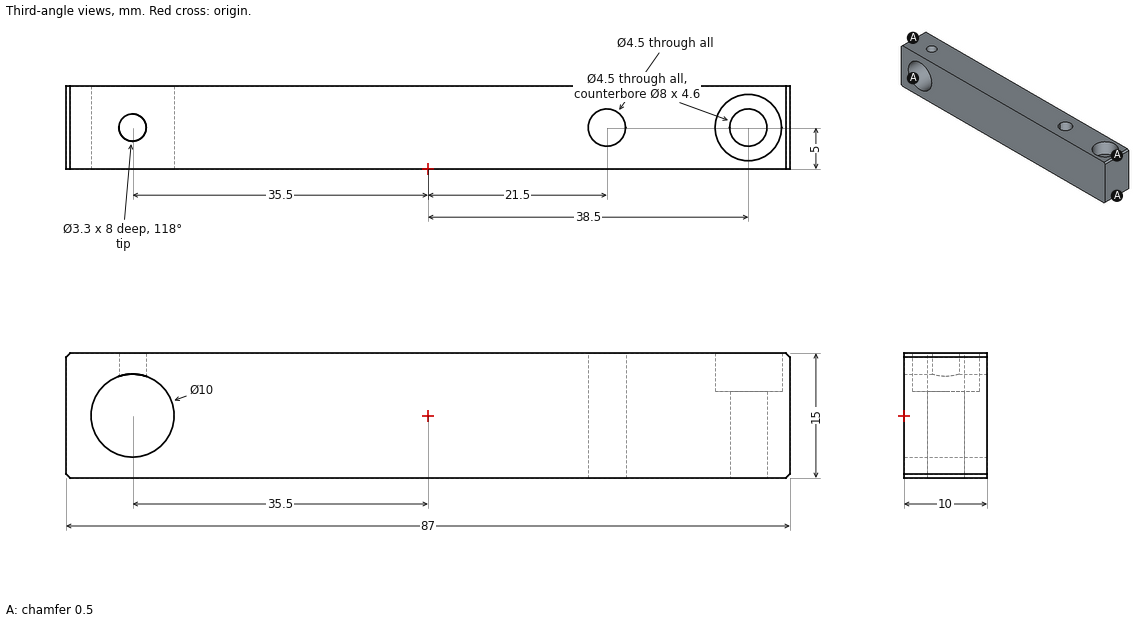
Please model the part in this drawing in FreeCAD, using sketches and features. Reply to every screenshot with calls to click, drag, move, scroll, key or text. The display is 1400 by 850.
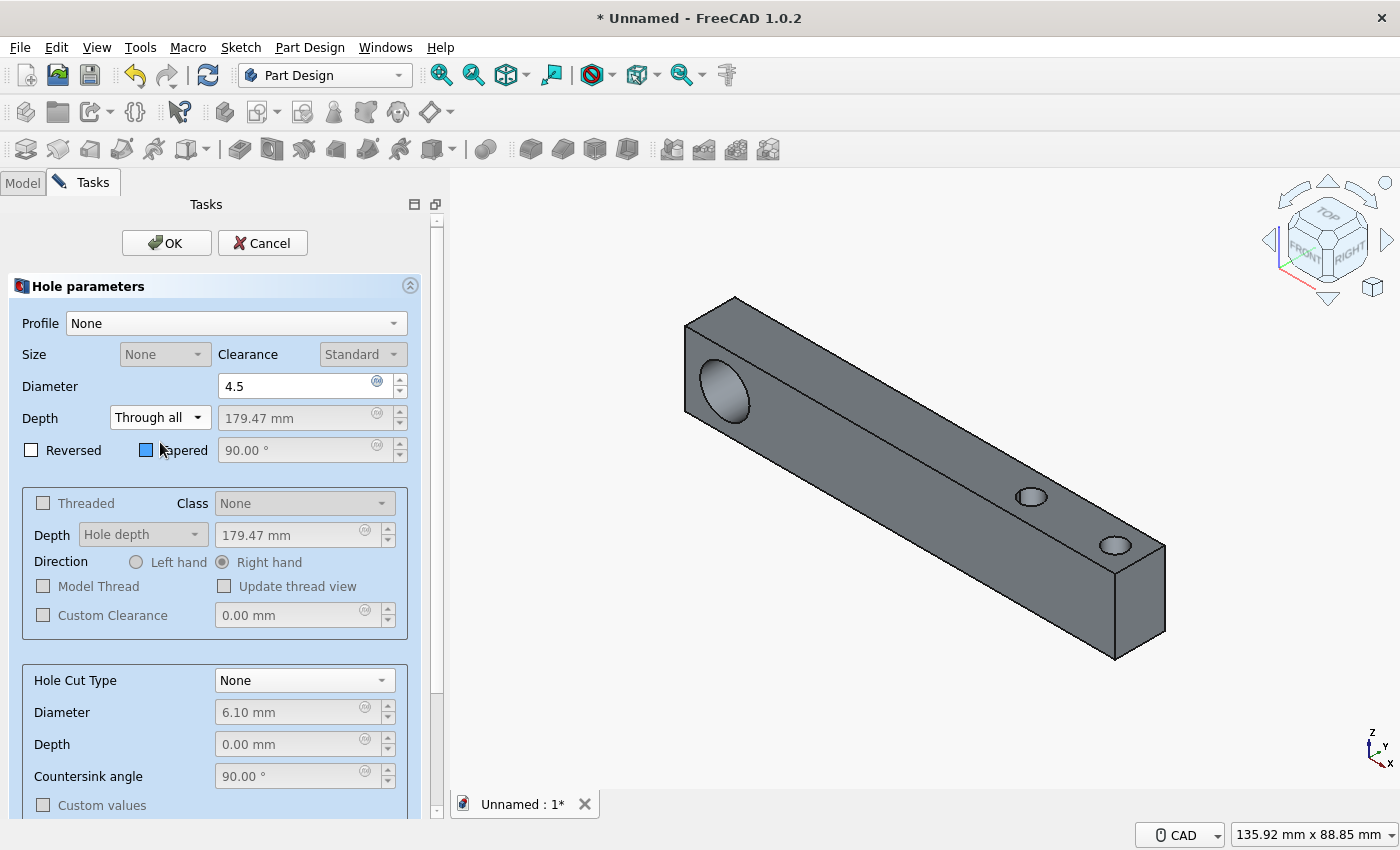
click(306, 680)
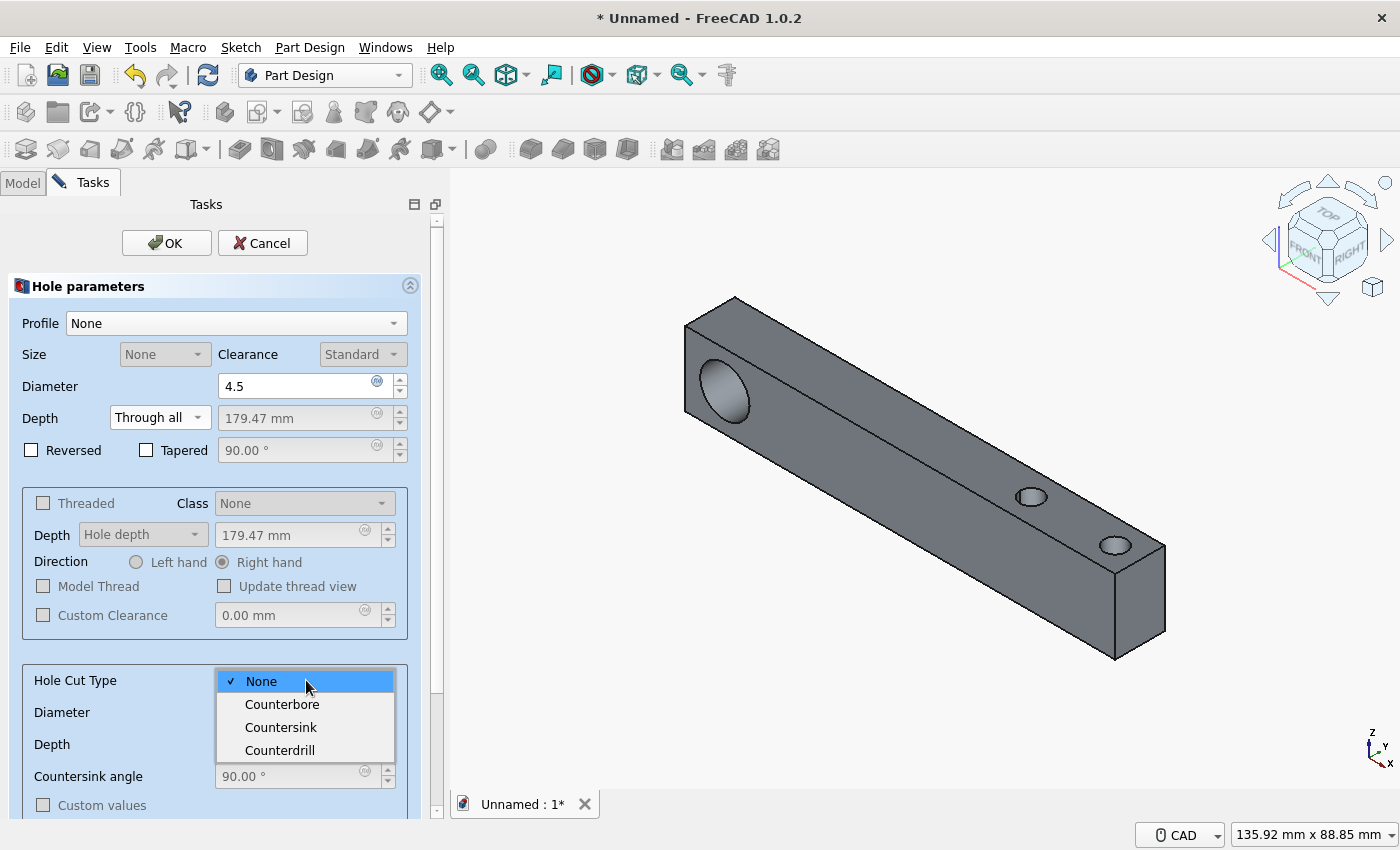
click(304, 704)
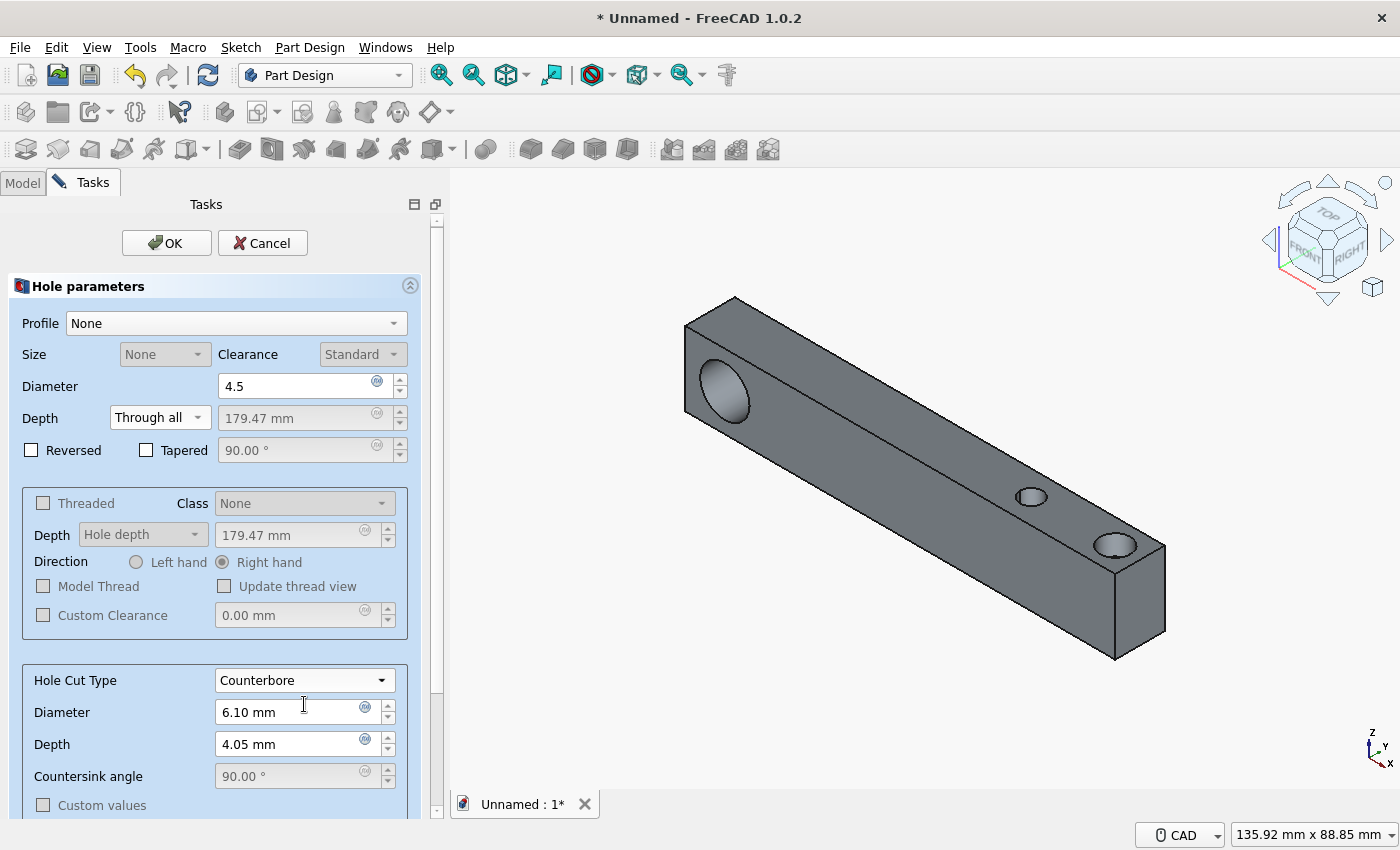
triple_click(298, 712)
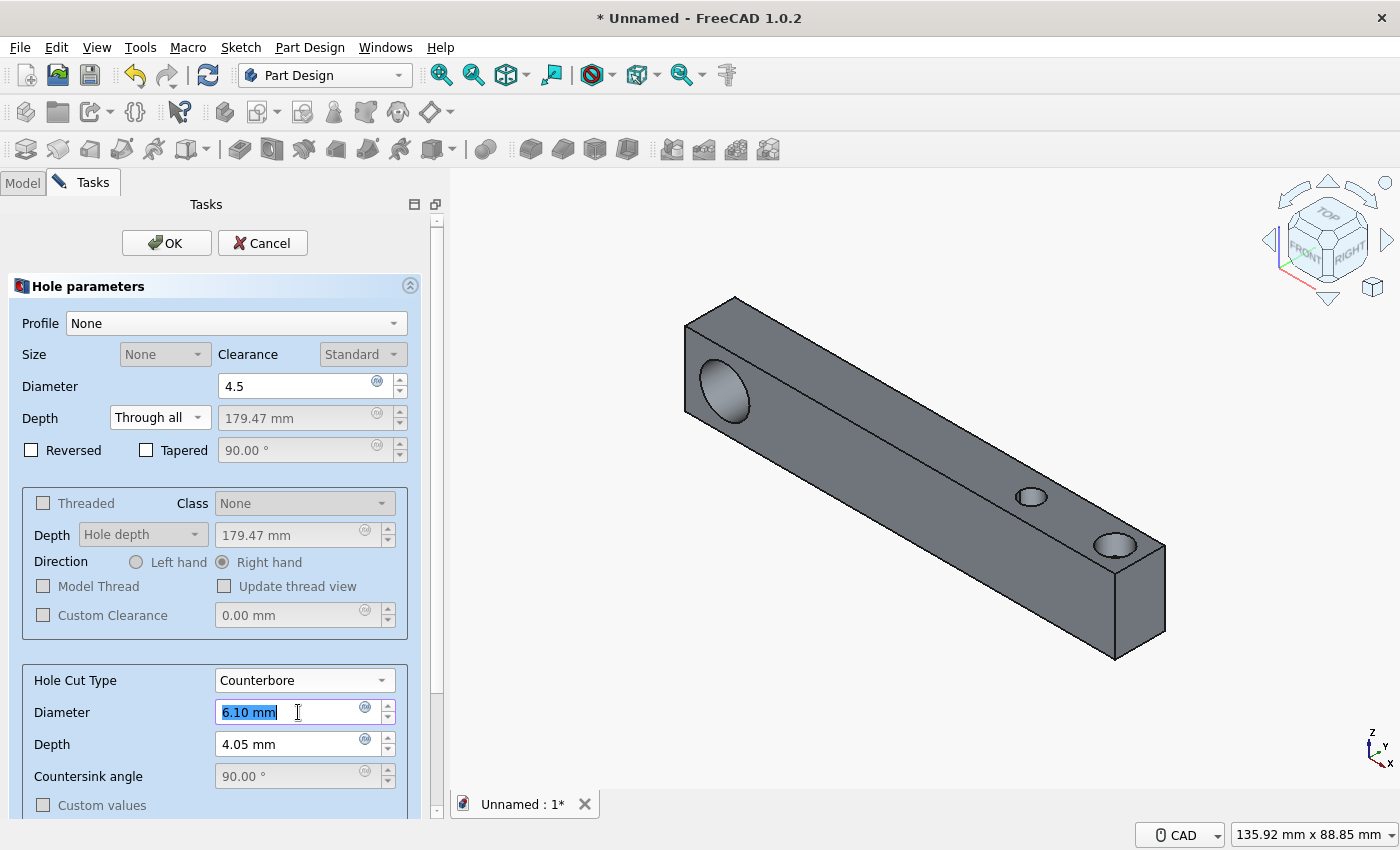
text(8)
key(Tab)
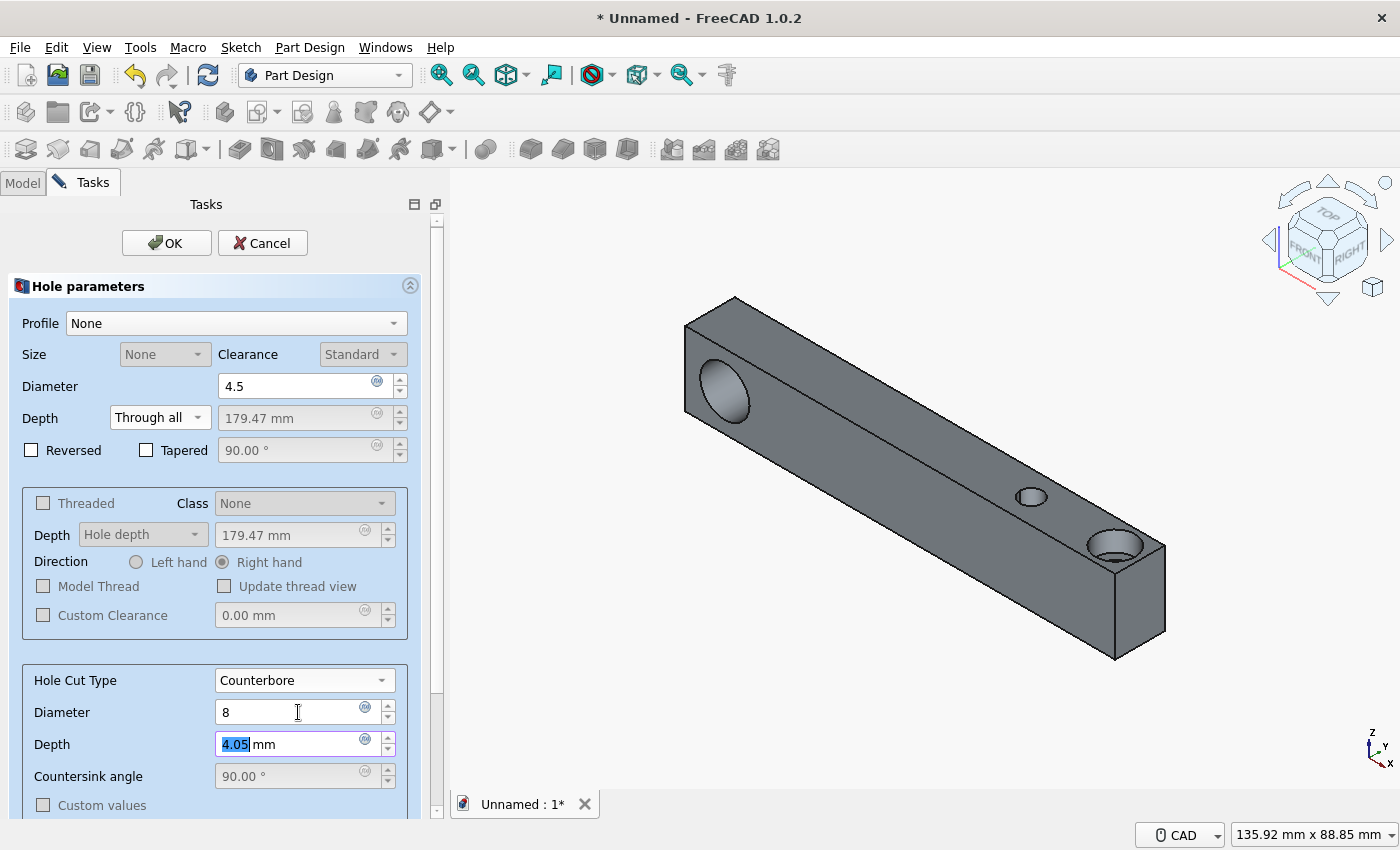
text(4.6)
key(Tab)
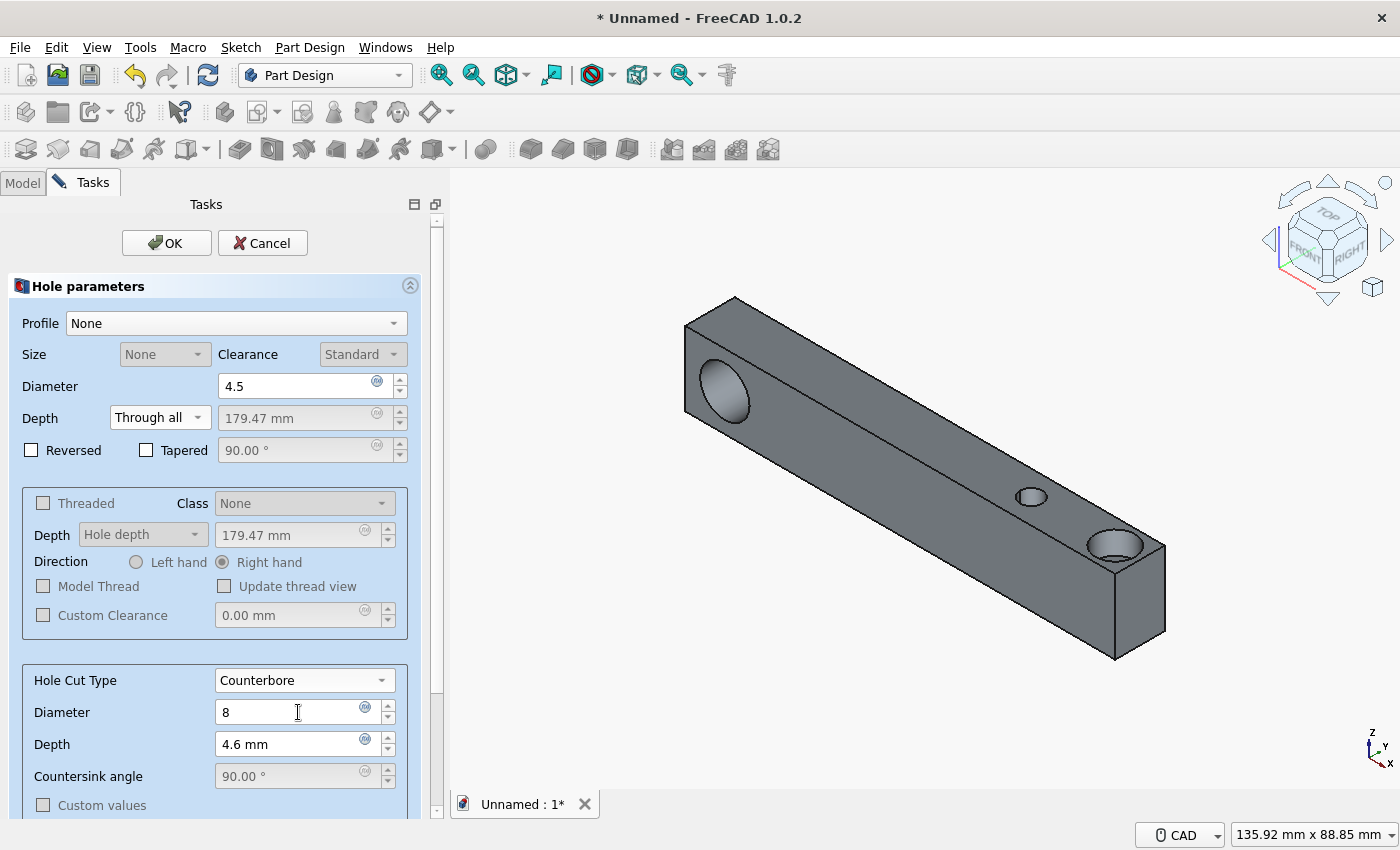
click(167, 243)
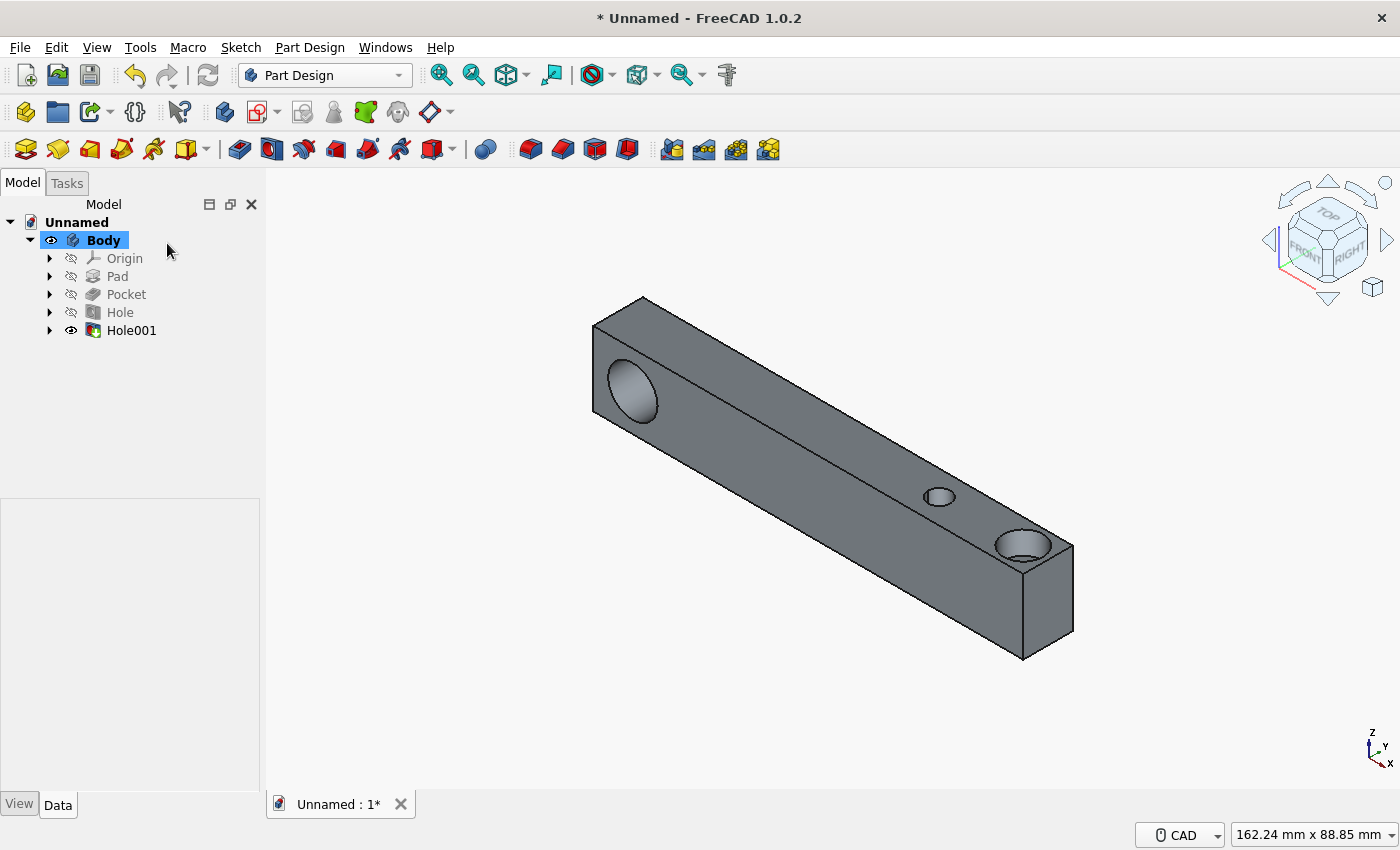
click(1048, 559)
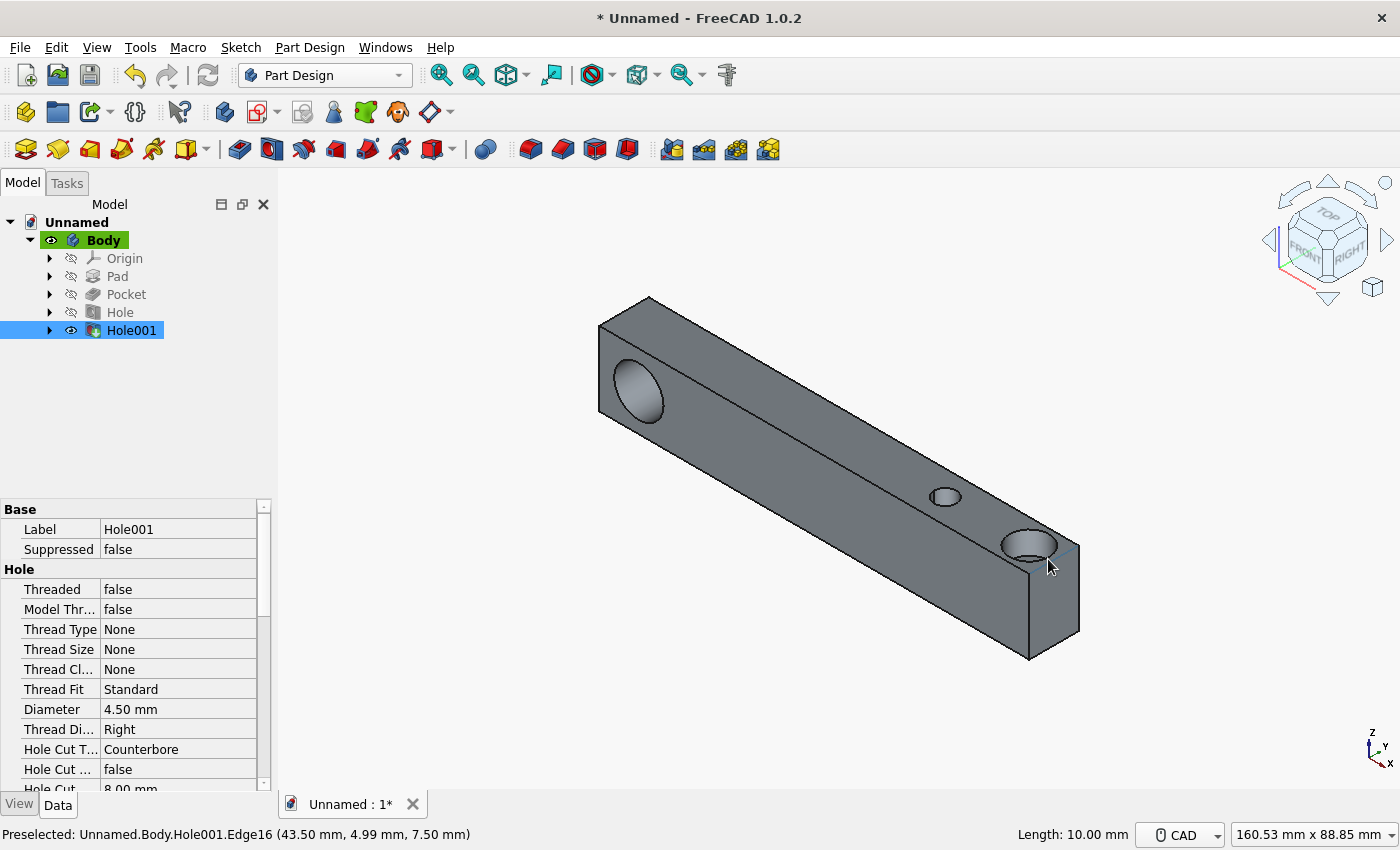
key(2)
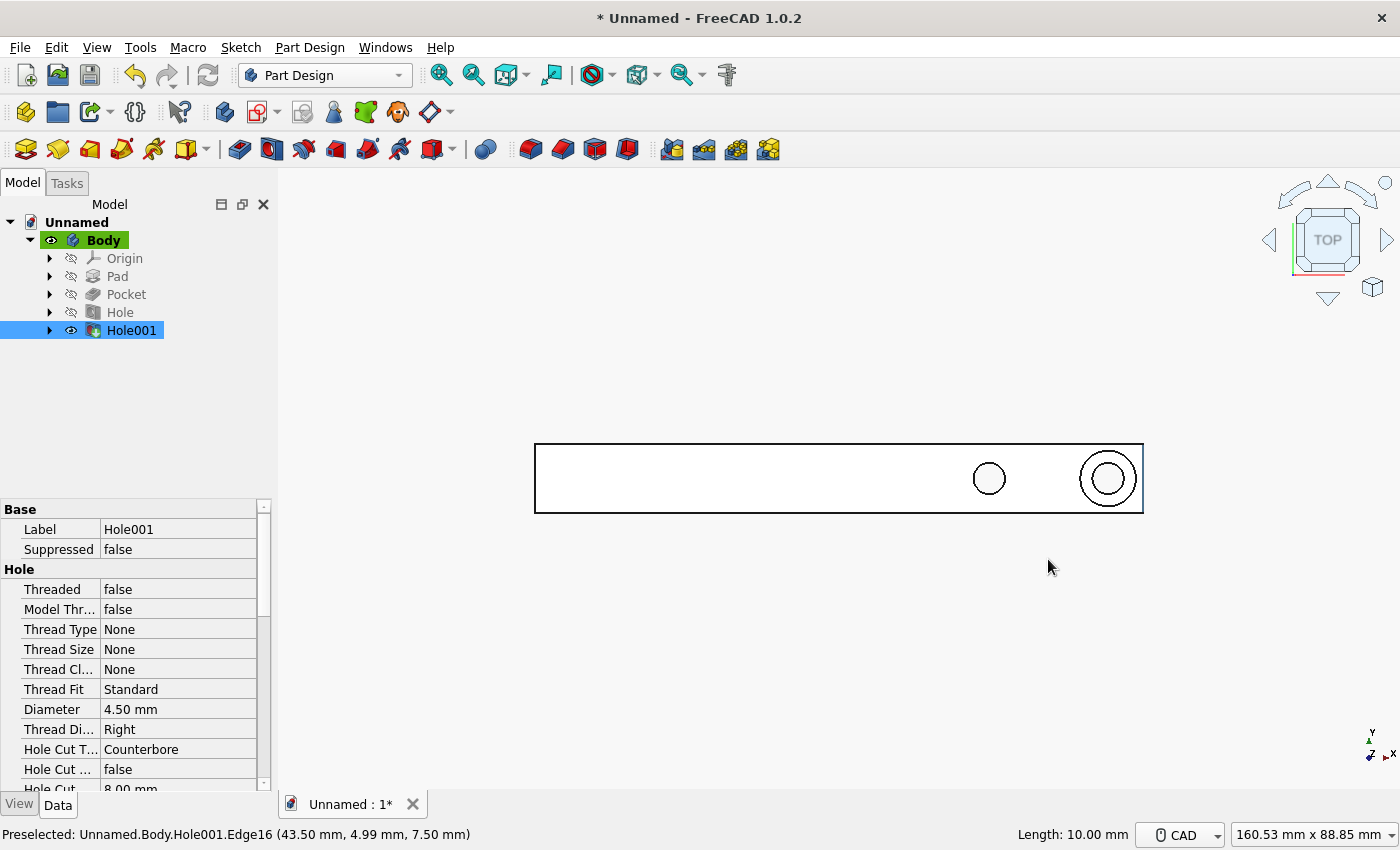
click(535, 477, ctrl)